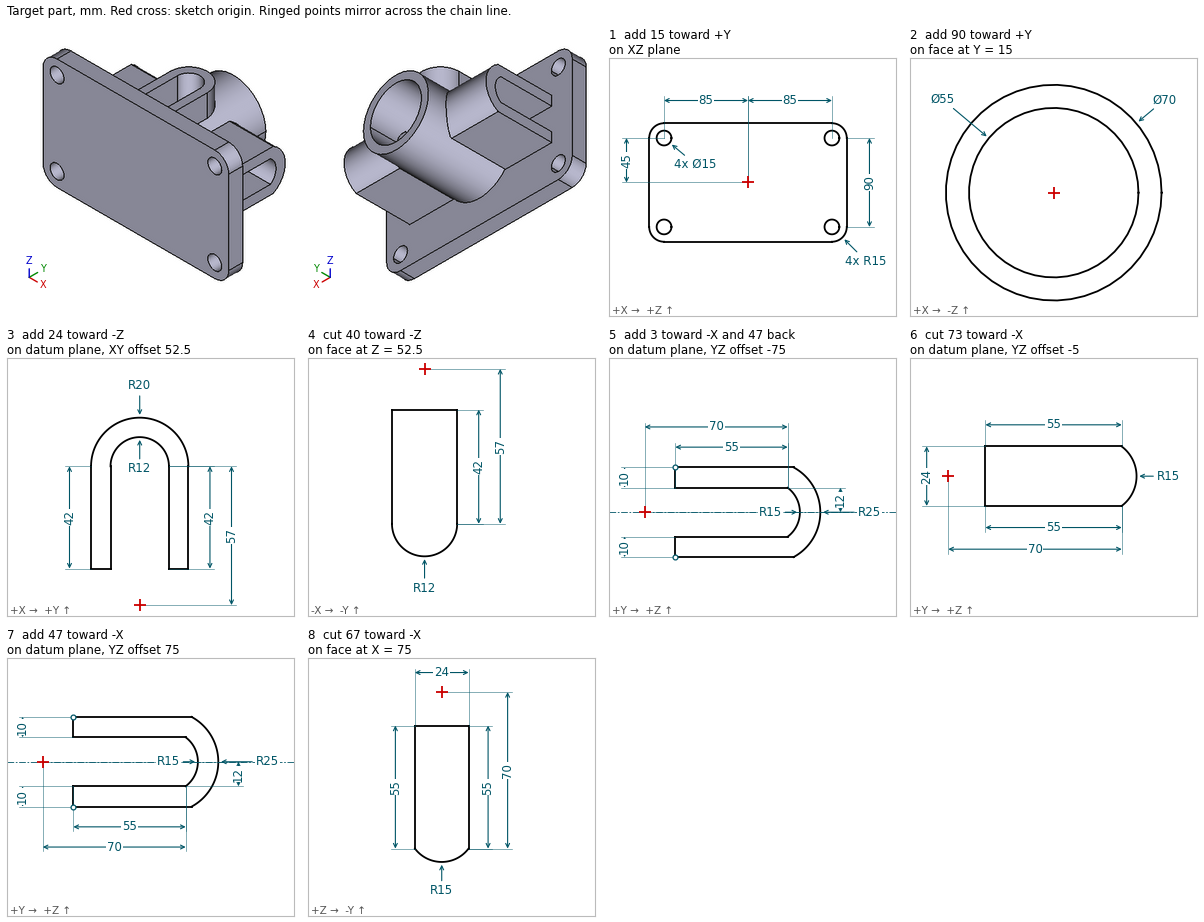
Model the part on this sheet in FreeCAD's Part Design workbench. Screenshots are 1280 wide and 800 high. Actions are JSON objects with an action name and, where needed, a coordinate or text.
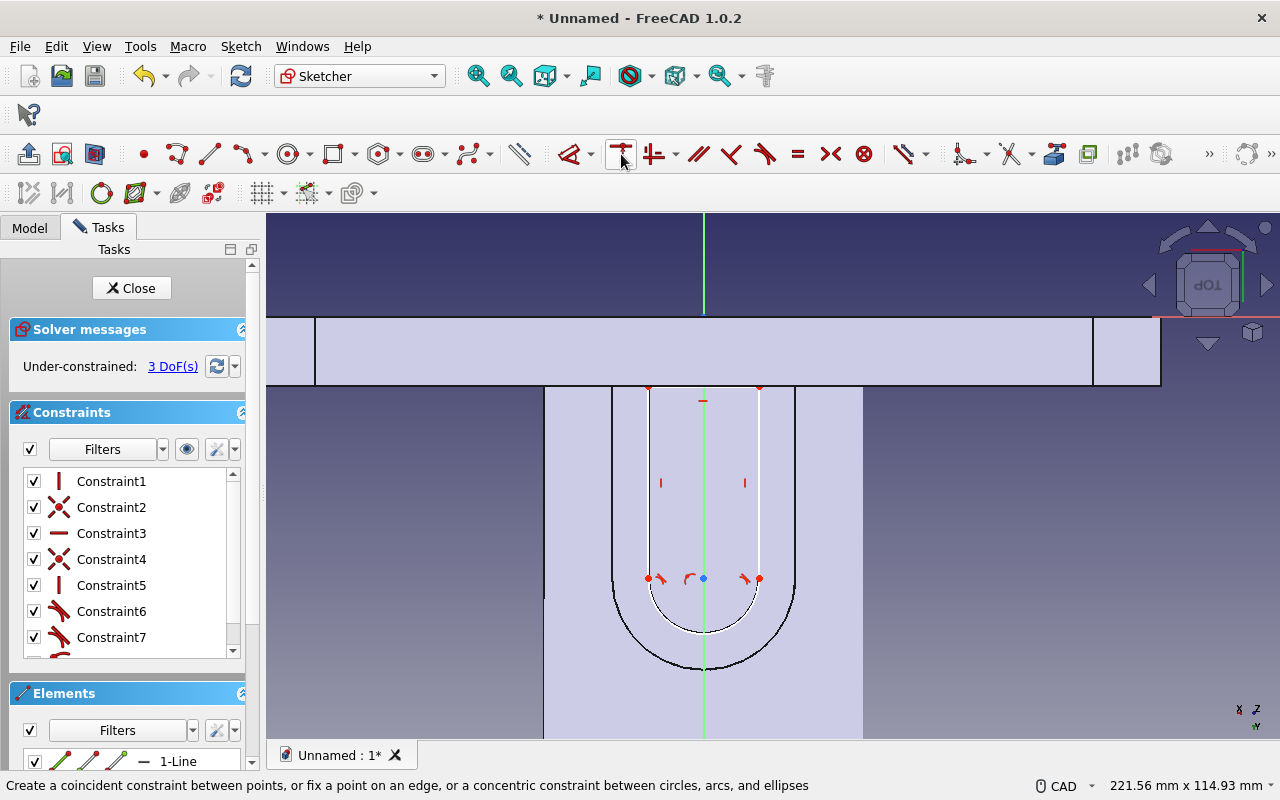
{"action": "left_click", "coordinate": [671, 623]}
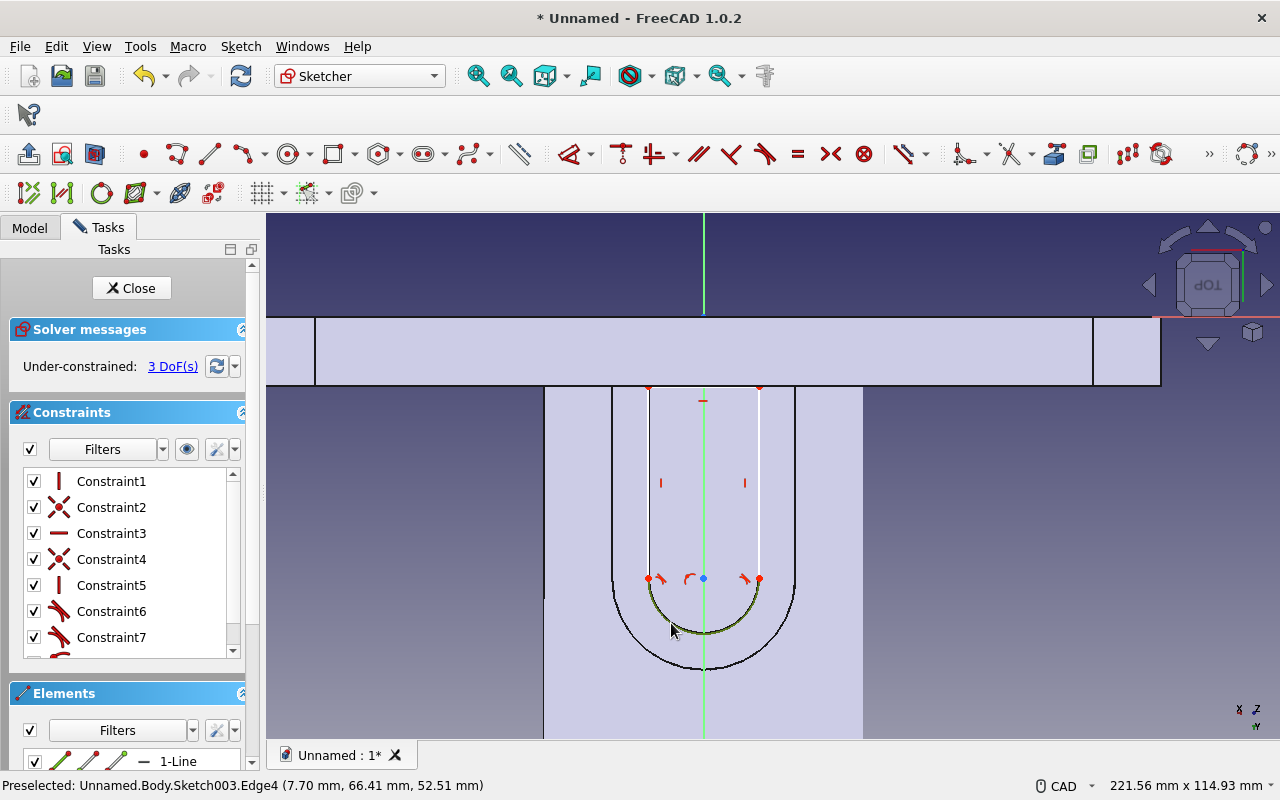
{"action": "key", "text": "k r"}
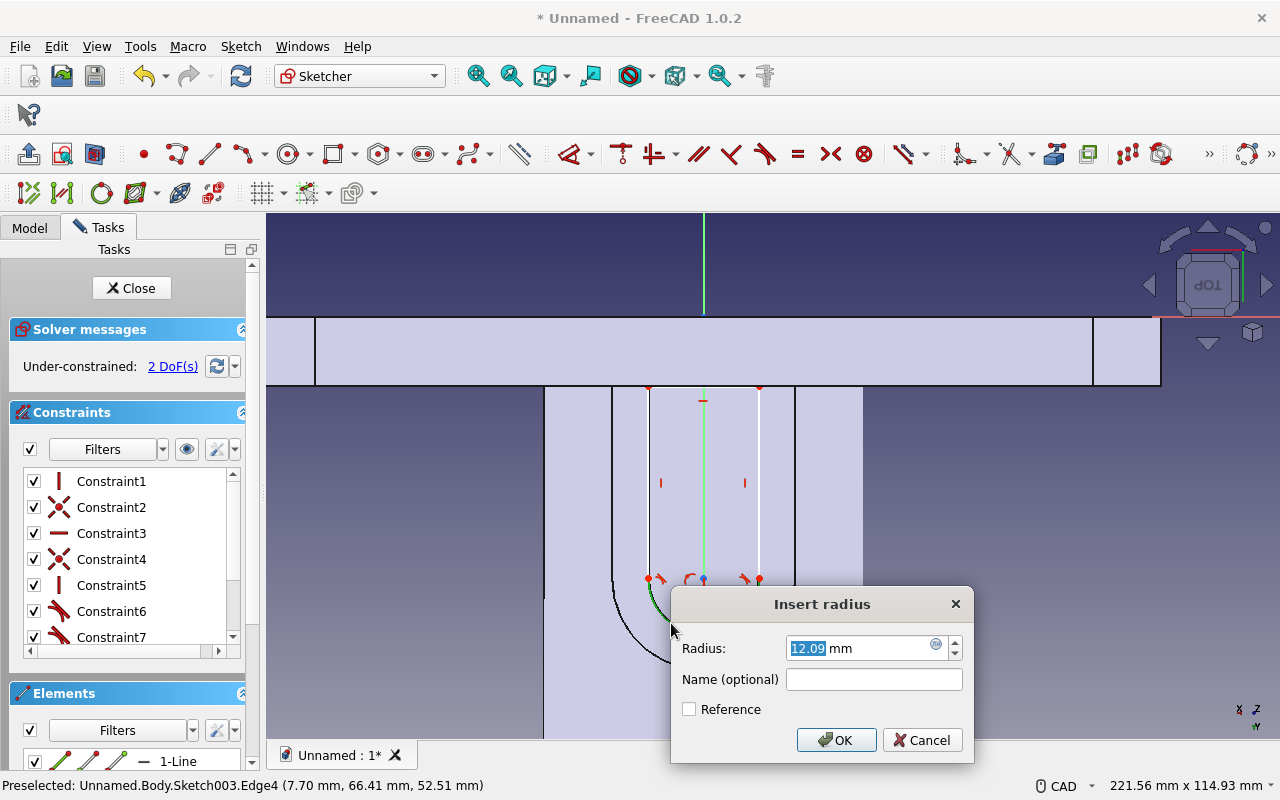
{"action": "type", "text": "12"}
{"action": "key", "text": "Return"}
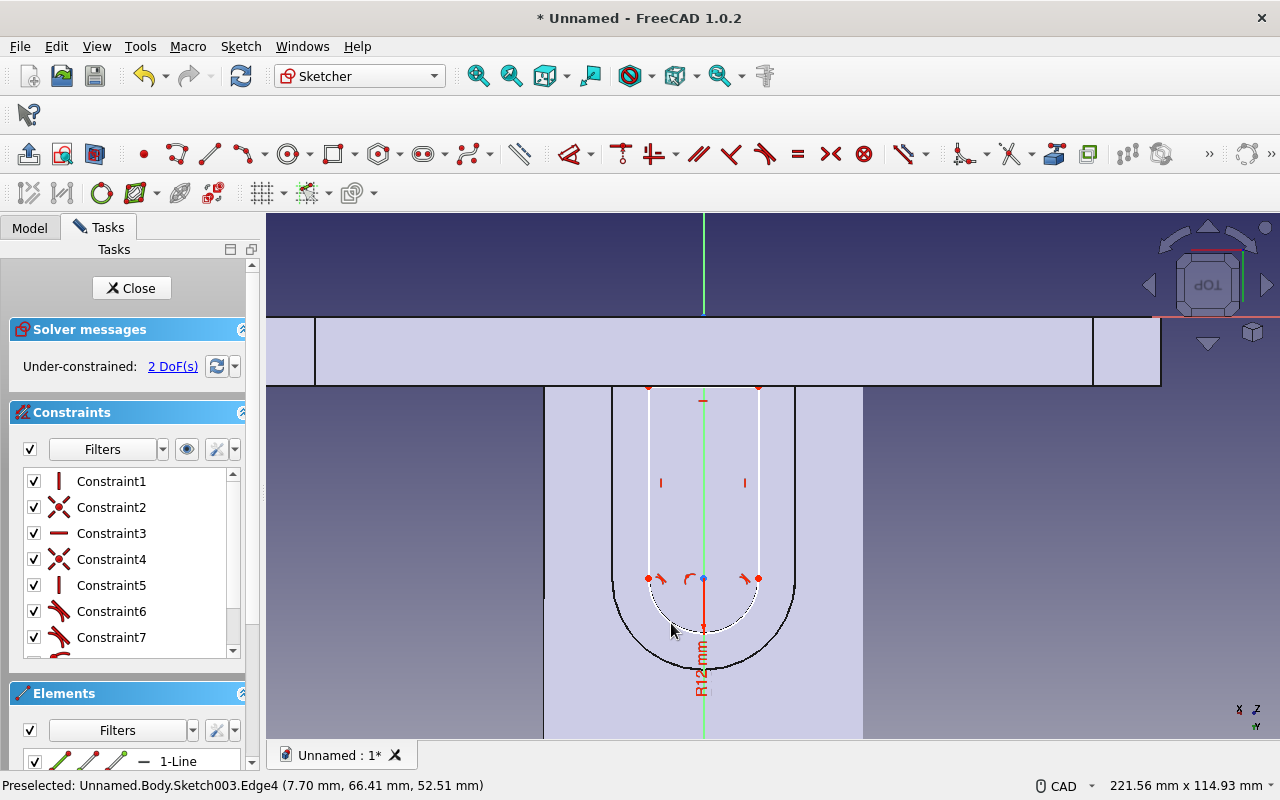
{"action": "left_click", "coordinate": [759, 521]}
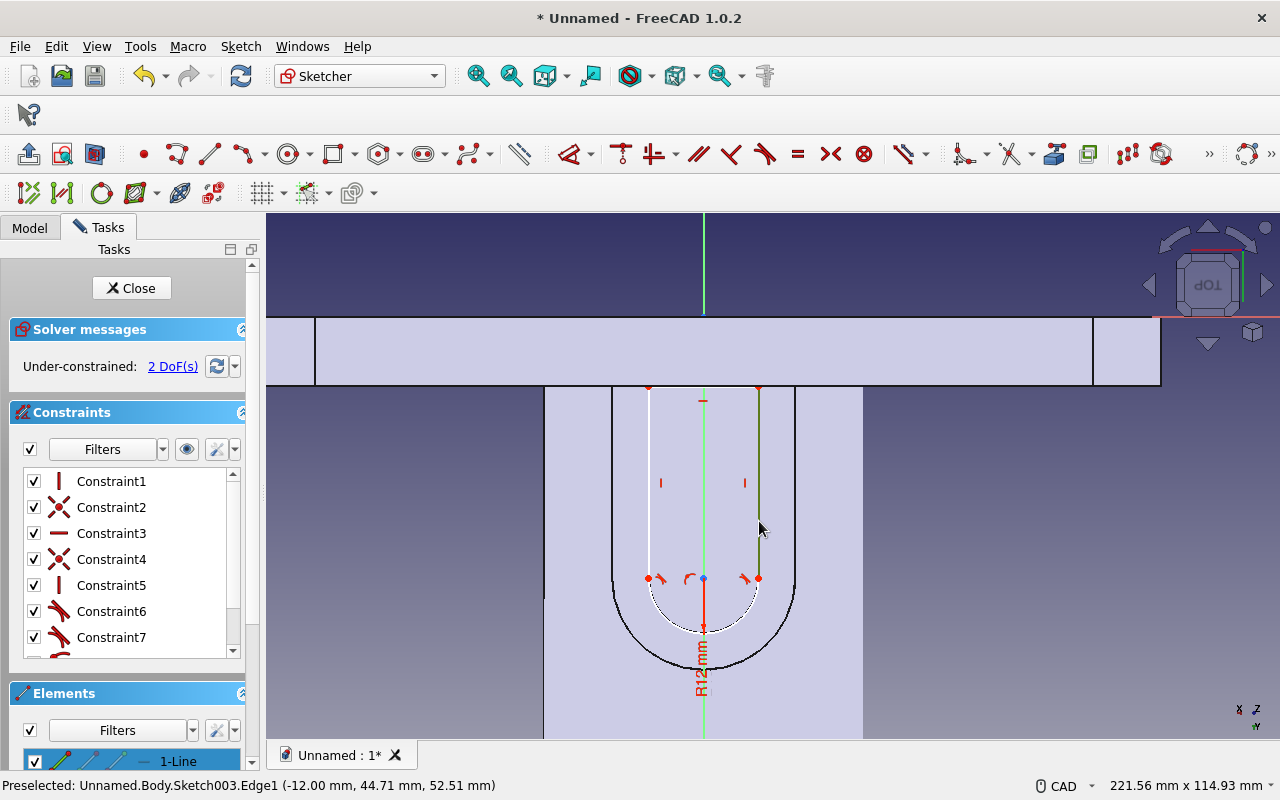
{"action": "key", "text": "i"}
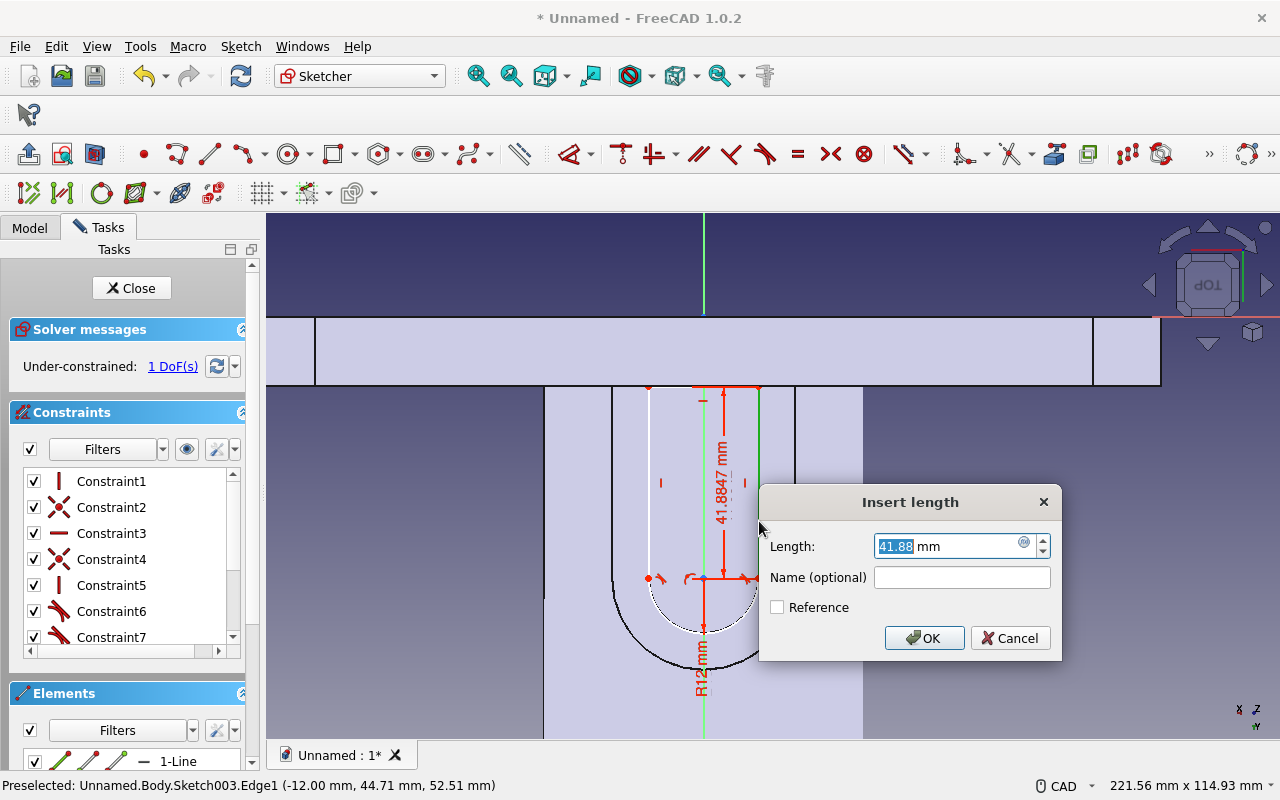
{"action": "type", "text": "42"}
{"action": "key", "text": "Return"}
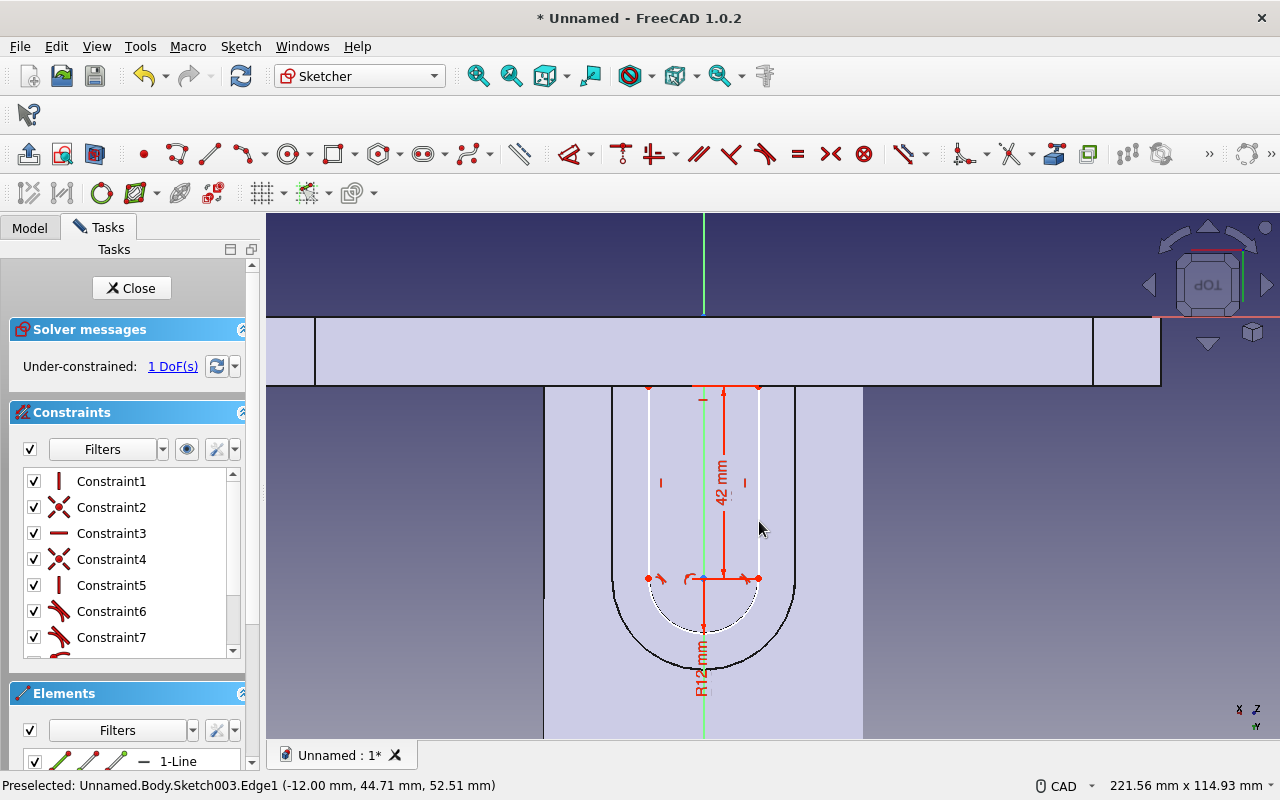
{"action": "left_click", "coordinate": [759, 579]}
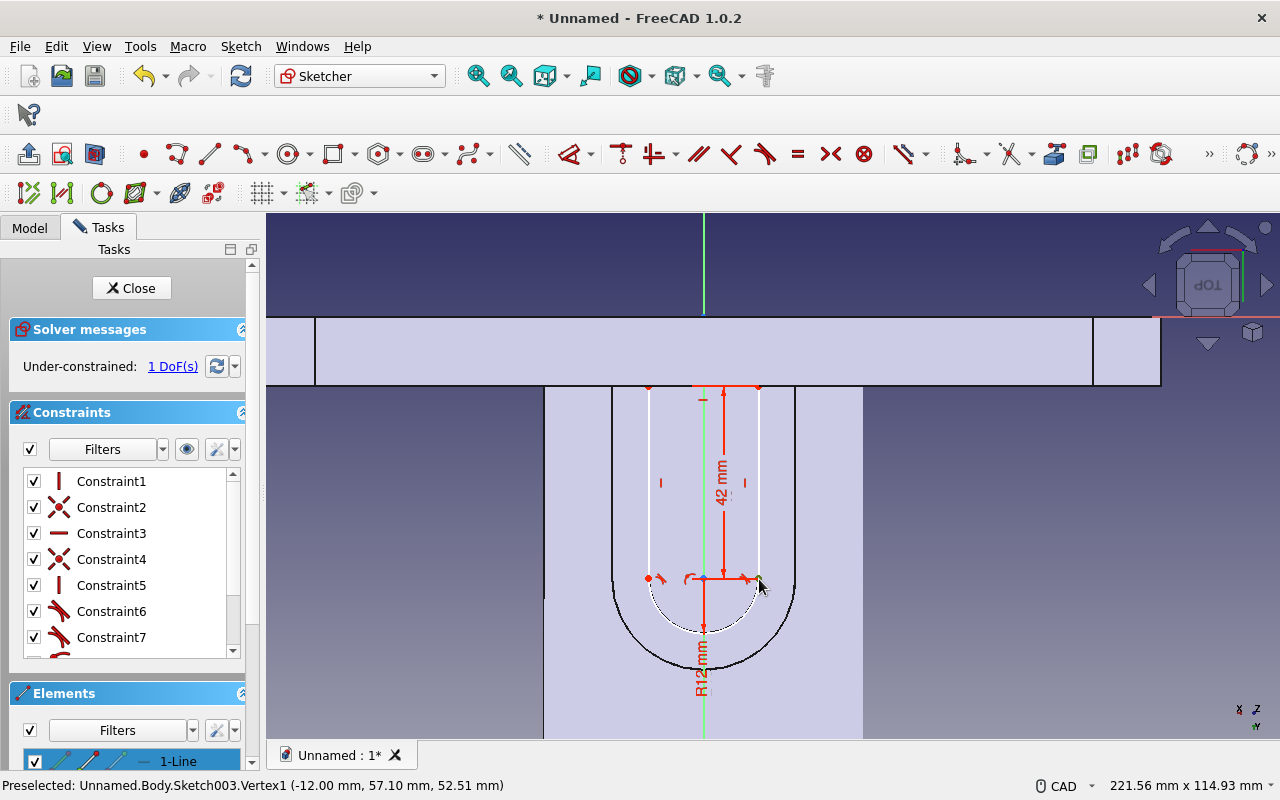
{"action": "key", "text": "i"}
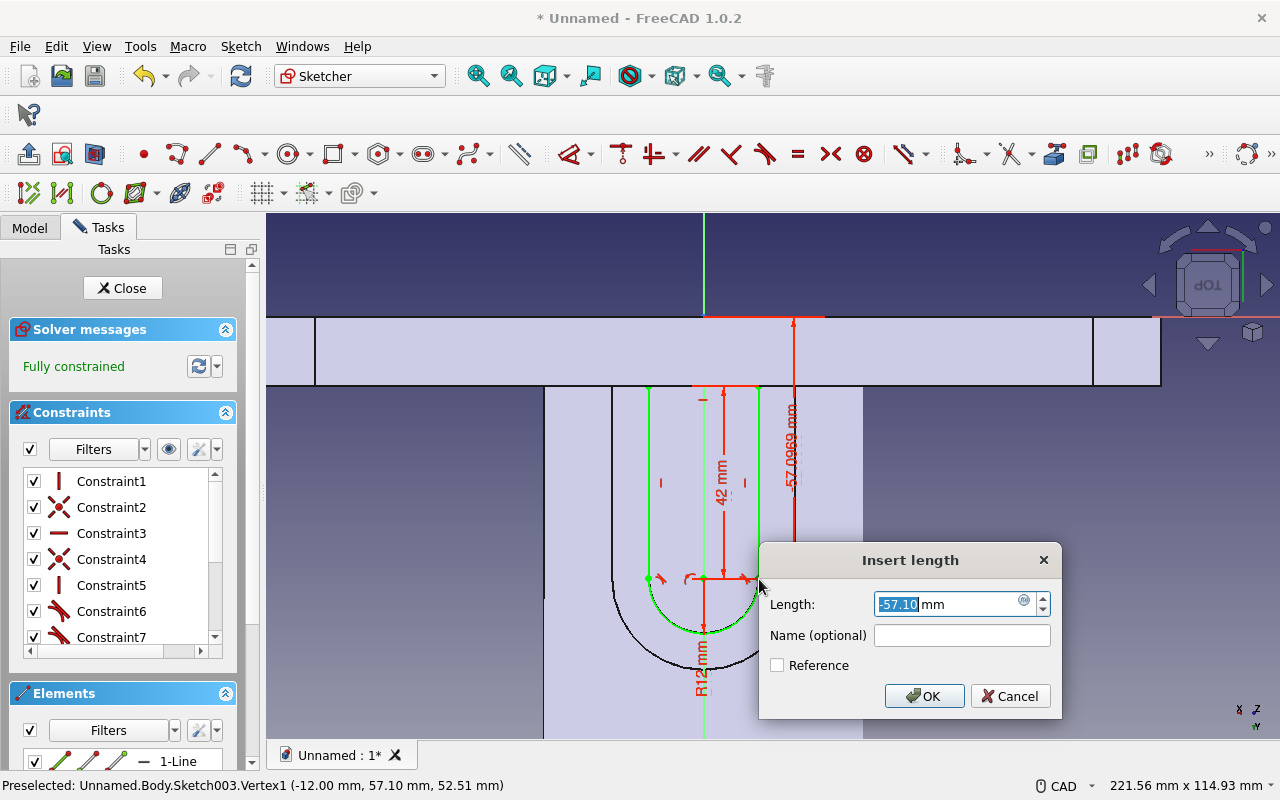
{"action": "type", "text": "-57"}
{"action": "key", "text": "Return"}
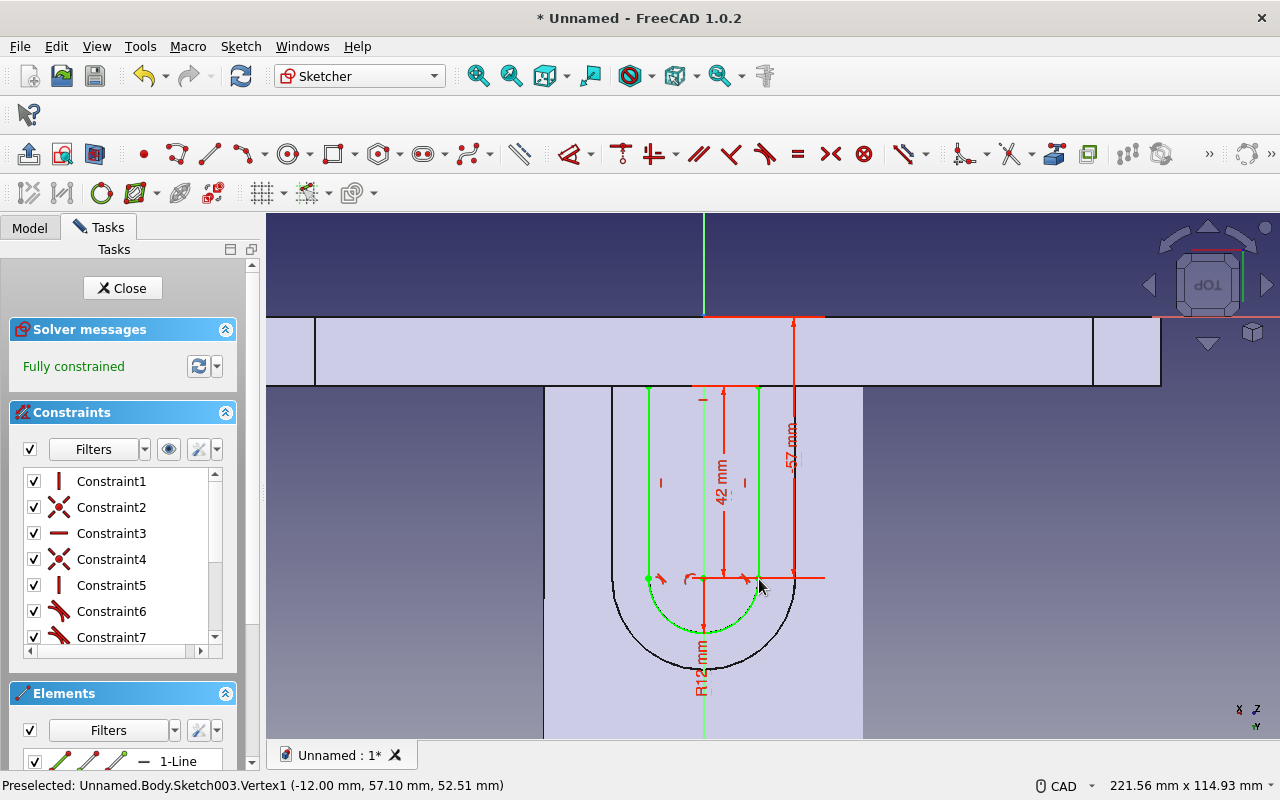
{"action": "left_click", "coordinate": [123, 288]}